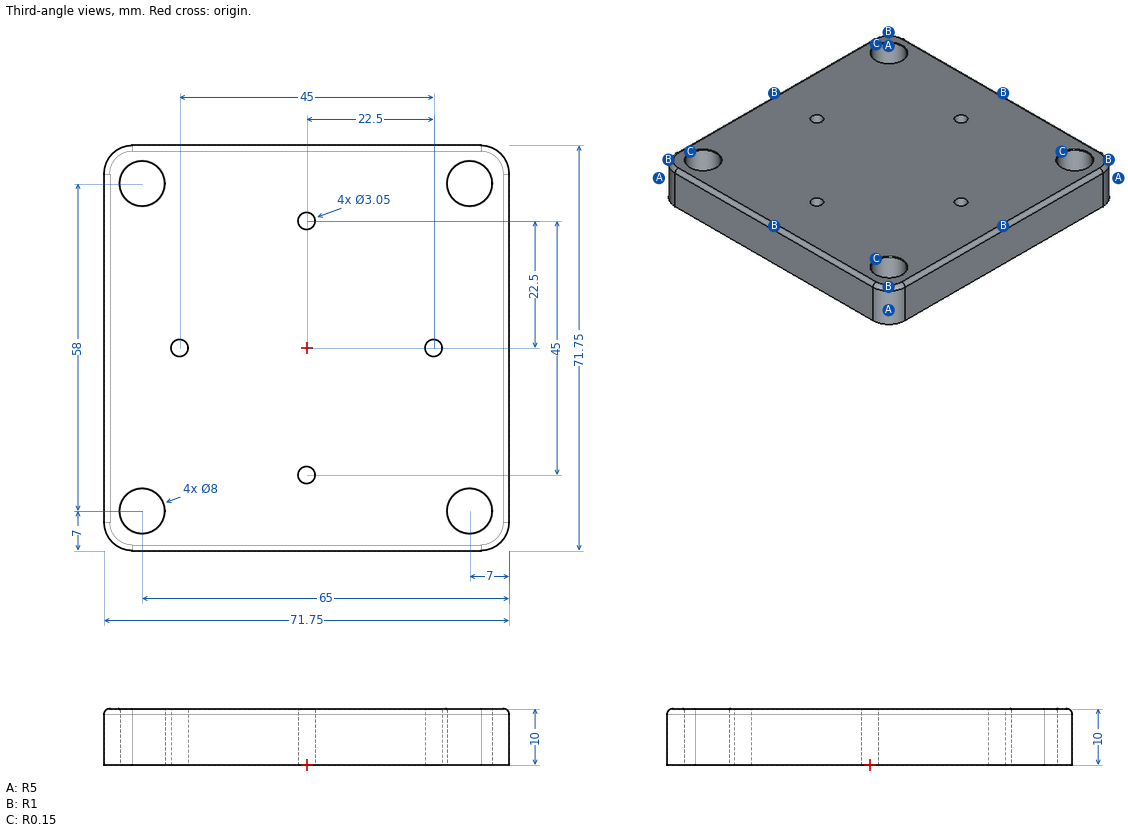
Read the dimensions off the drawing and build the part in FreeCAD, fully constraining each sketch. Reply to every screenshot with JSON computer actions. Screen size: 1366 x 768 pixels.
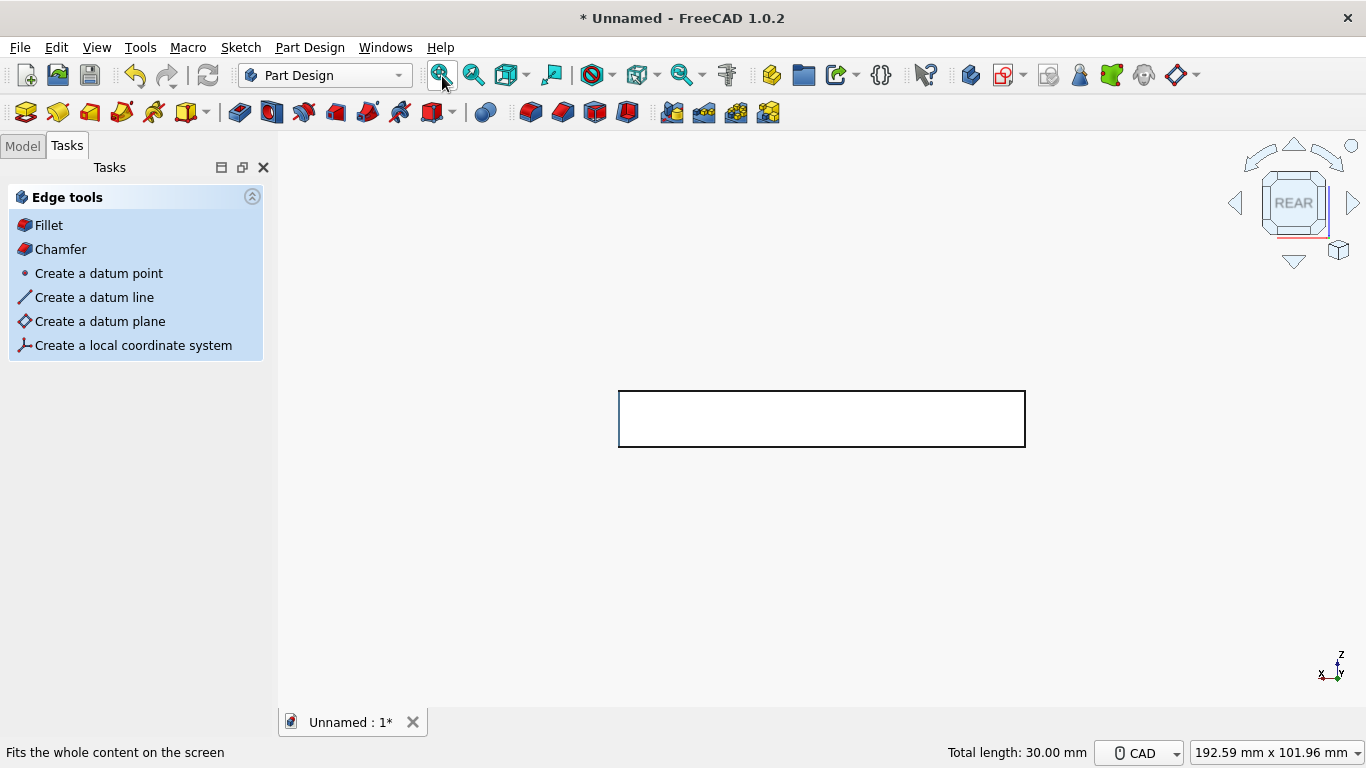
{"action": "left_click", "coordinate": [1025, 418], "text": "ctrl"}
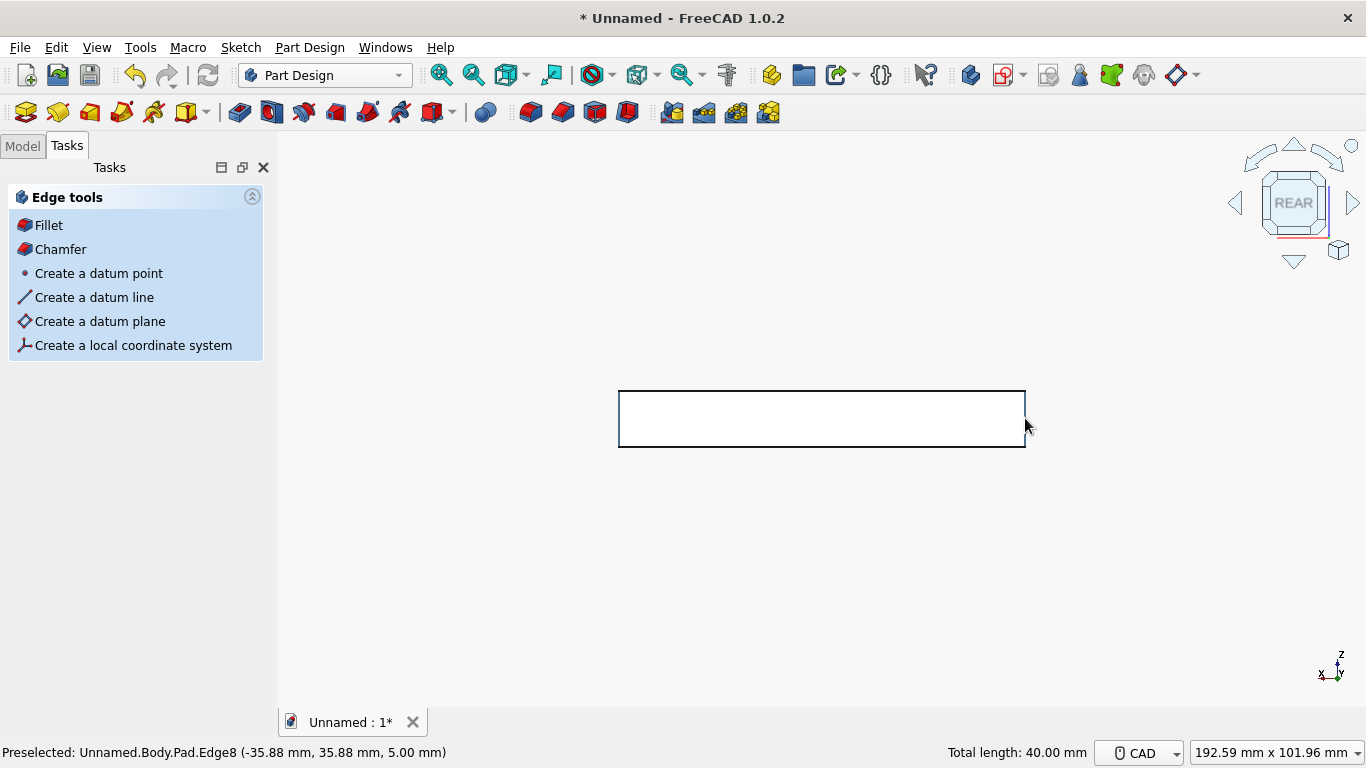
{"action": "left_click", "coordinate": [532, 112]}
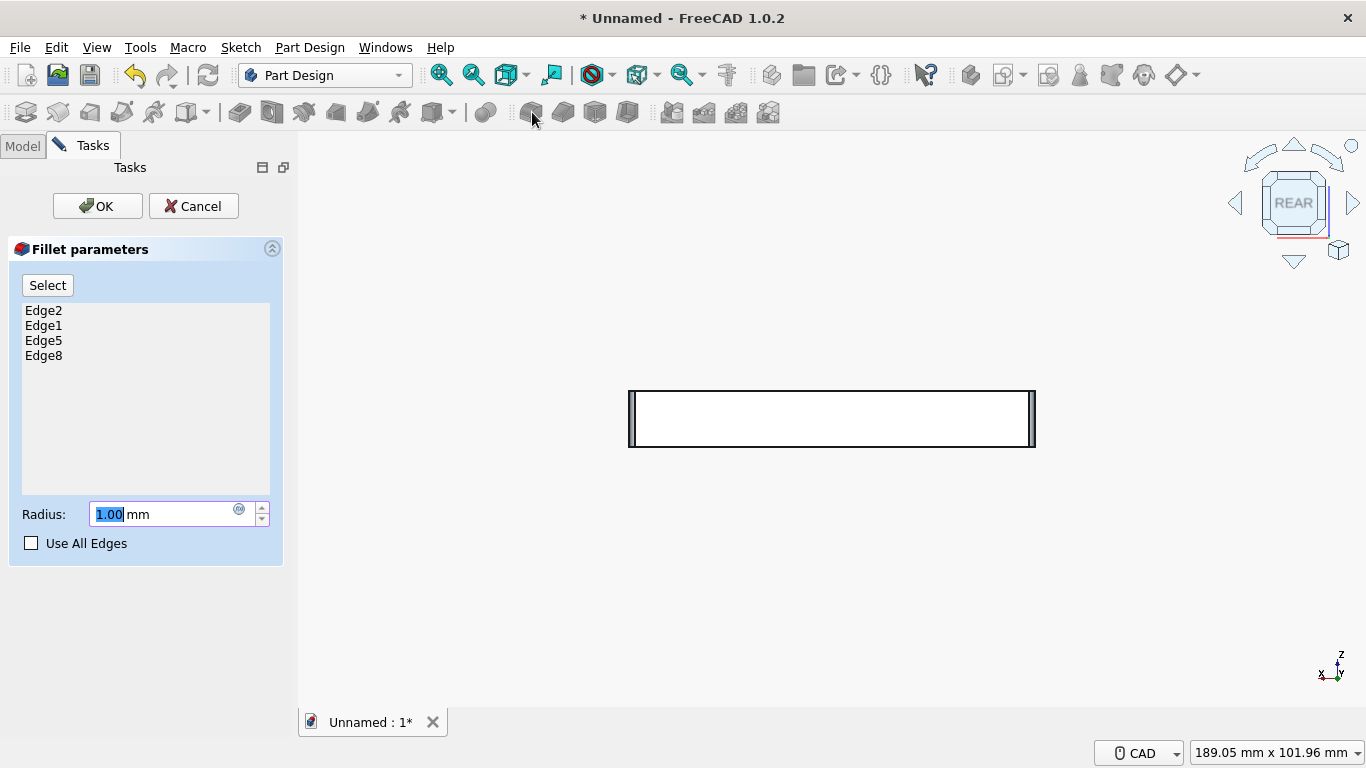
{"action": "type", "text": "5"}
{"action": "key", "text": "Tab"}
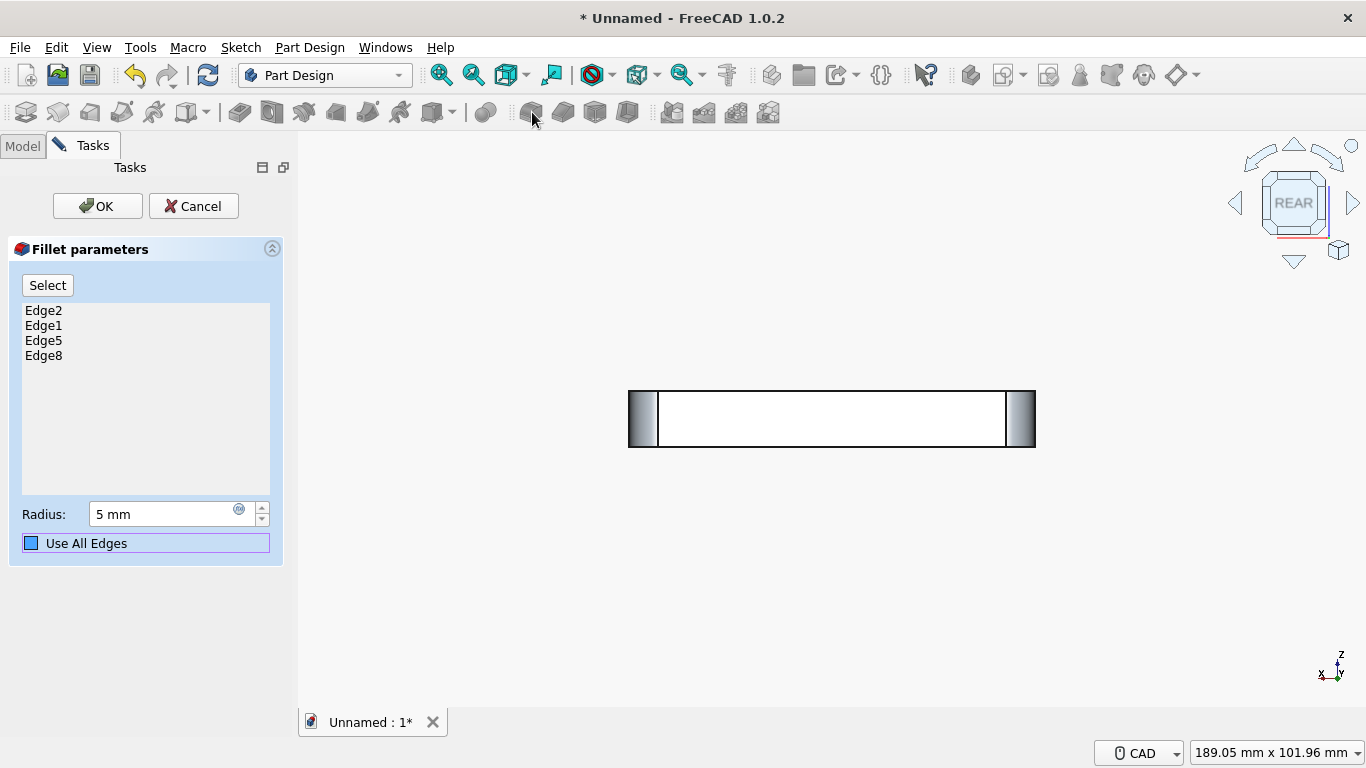
{"action": "left_click", "coordinate": [98, 206]}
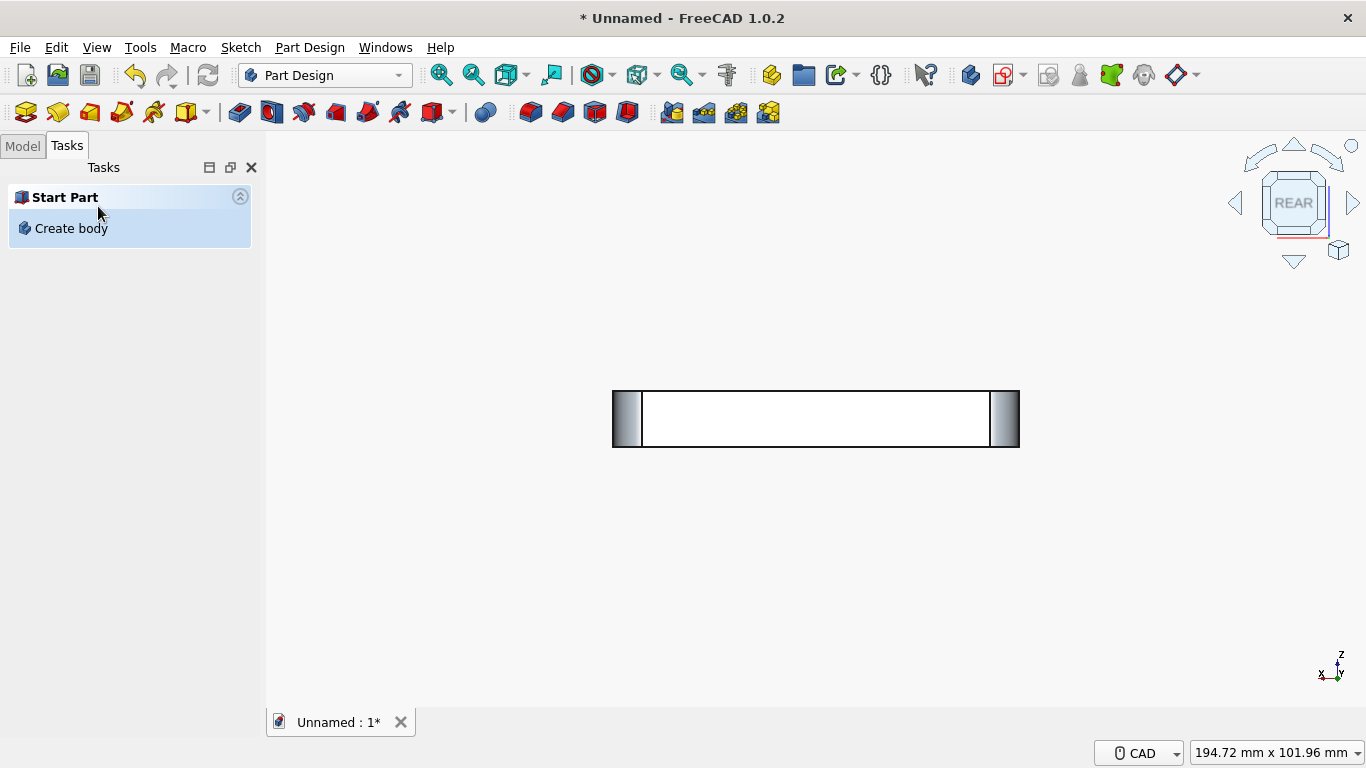
{"action": "left_click", "coordinate": [442, 76]}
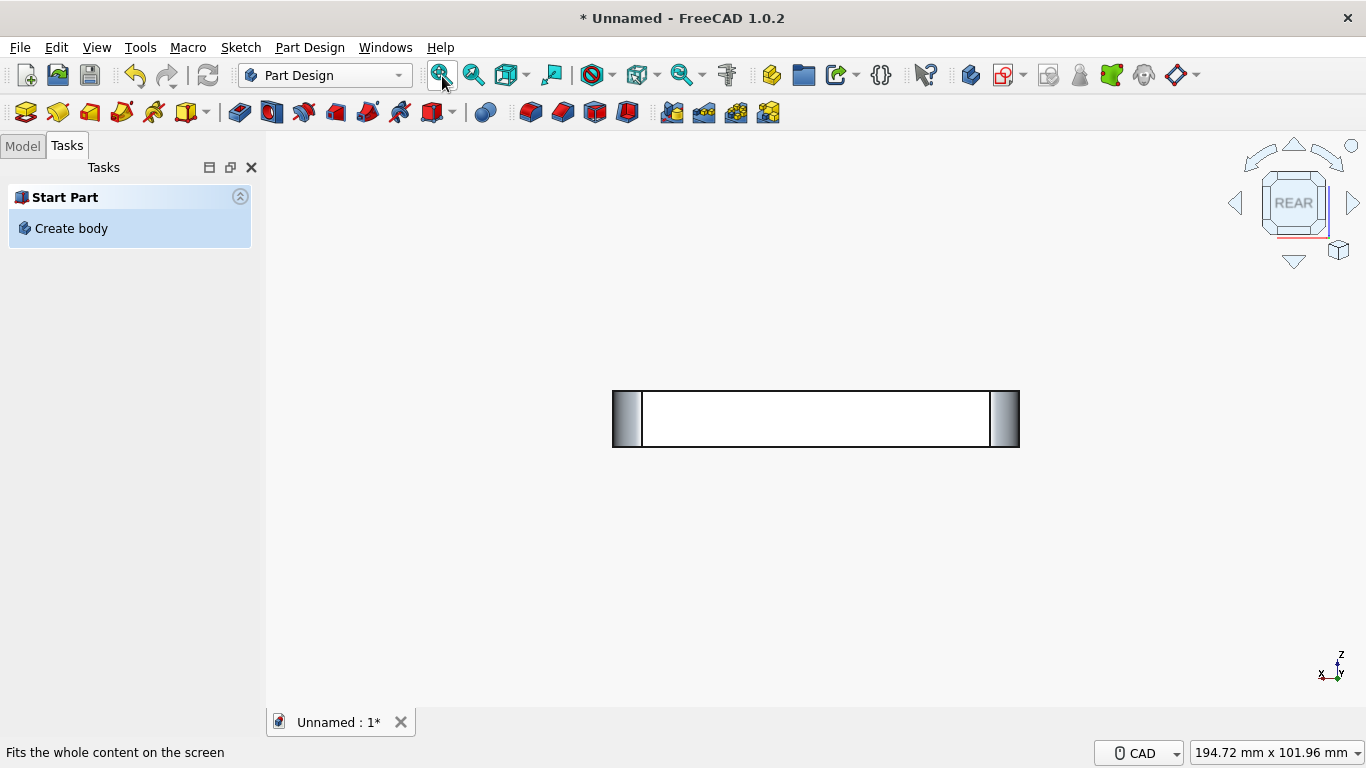
{"action": "left_click", "coordinate": [816, 390]}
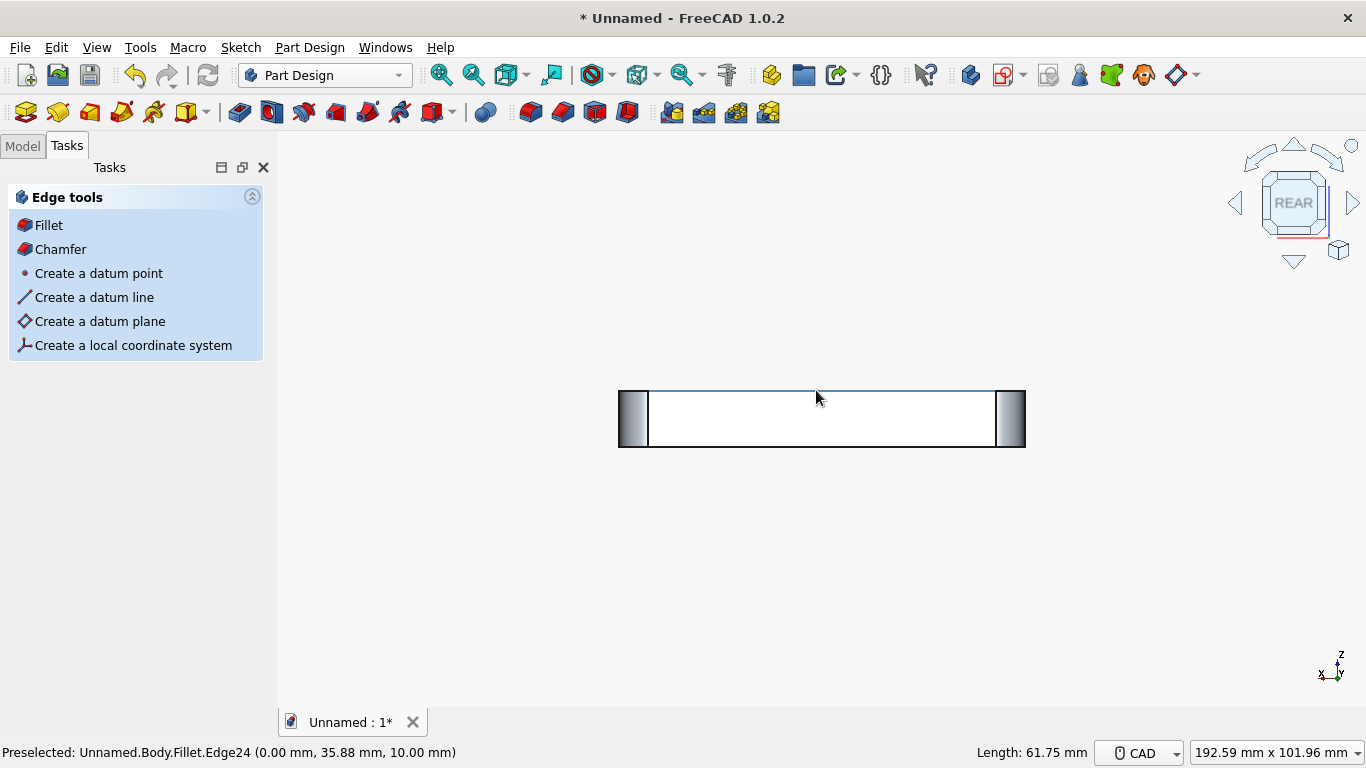
{"action": "left_click", "coordinate": [1016, 390], "text": "ctrl"}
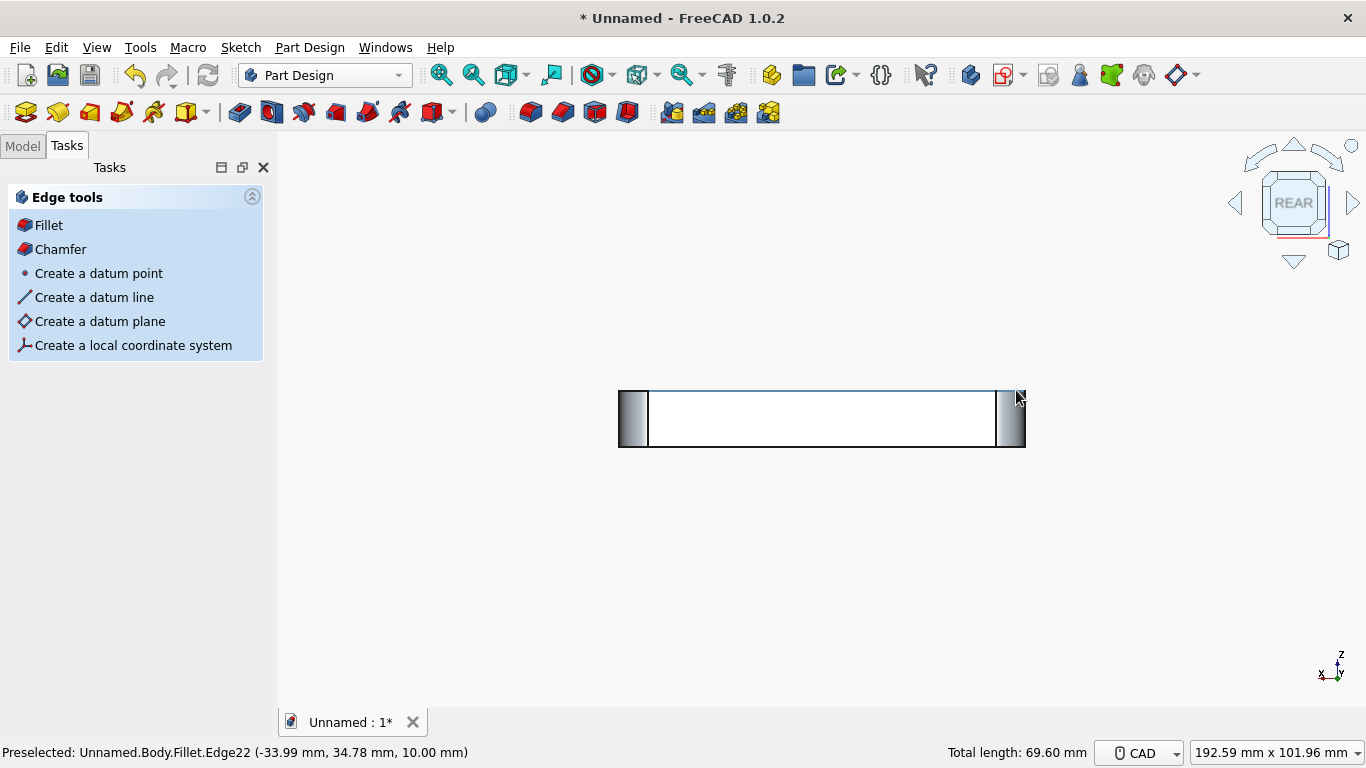
{"action": "left_click", "coordinate": [628, 390], "text": "ctrl"}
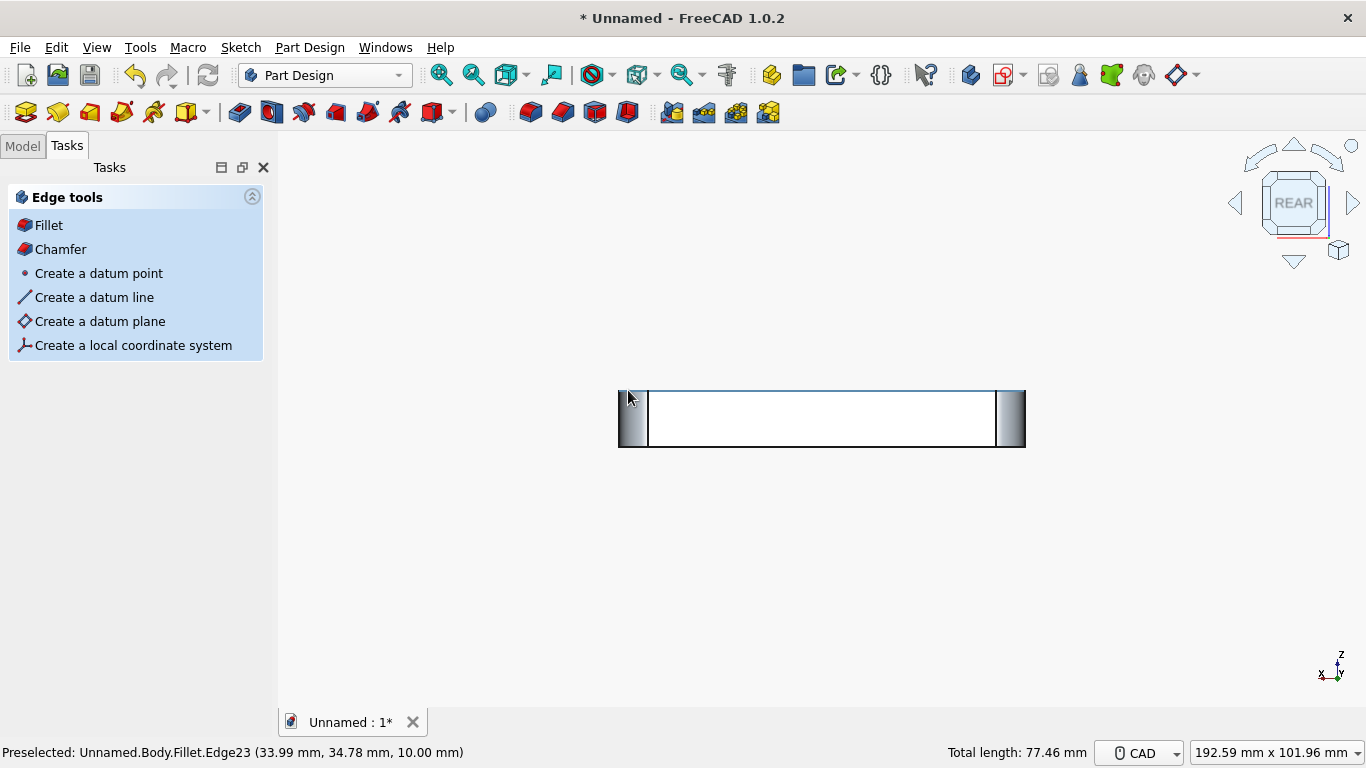
{"action": "key", "text": "0"}